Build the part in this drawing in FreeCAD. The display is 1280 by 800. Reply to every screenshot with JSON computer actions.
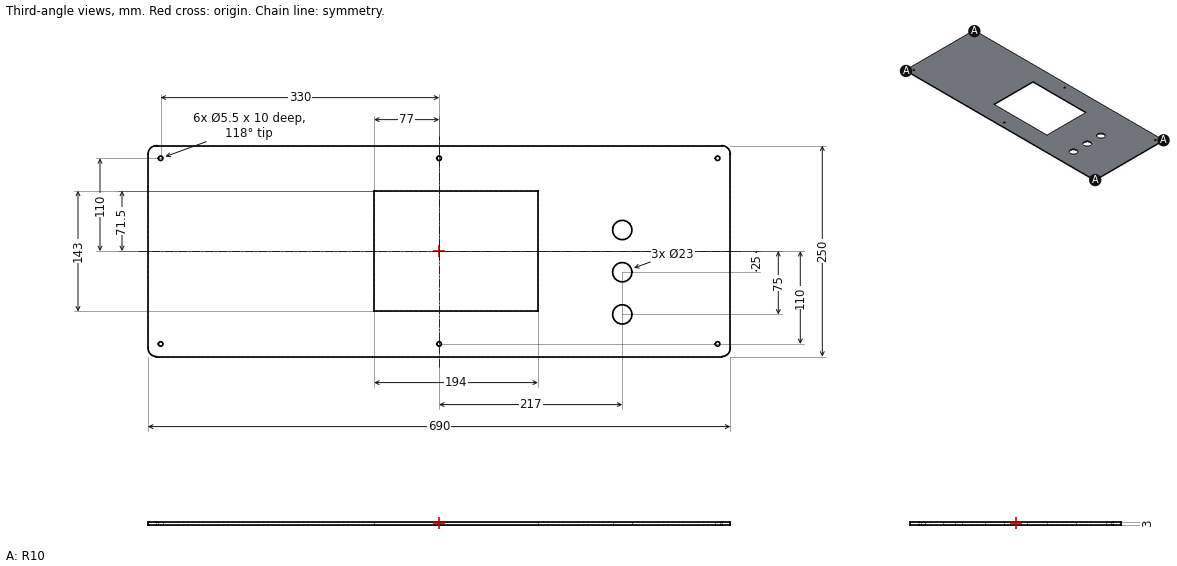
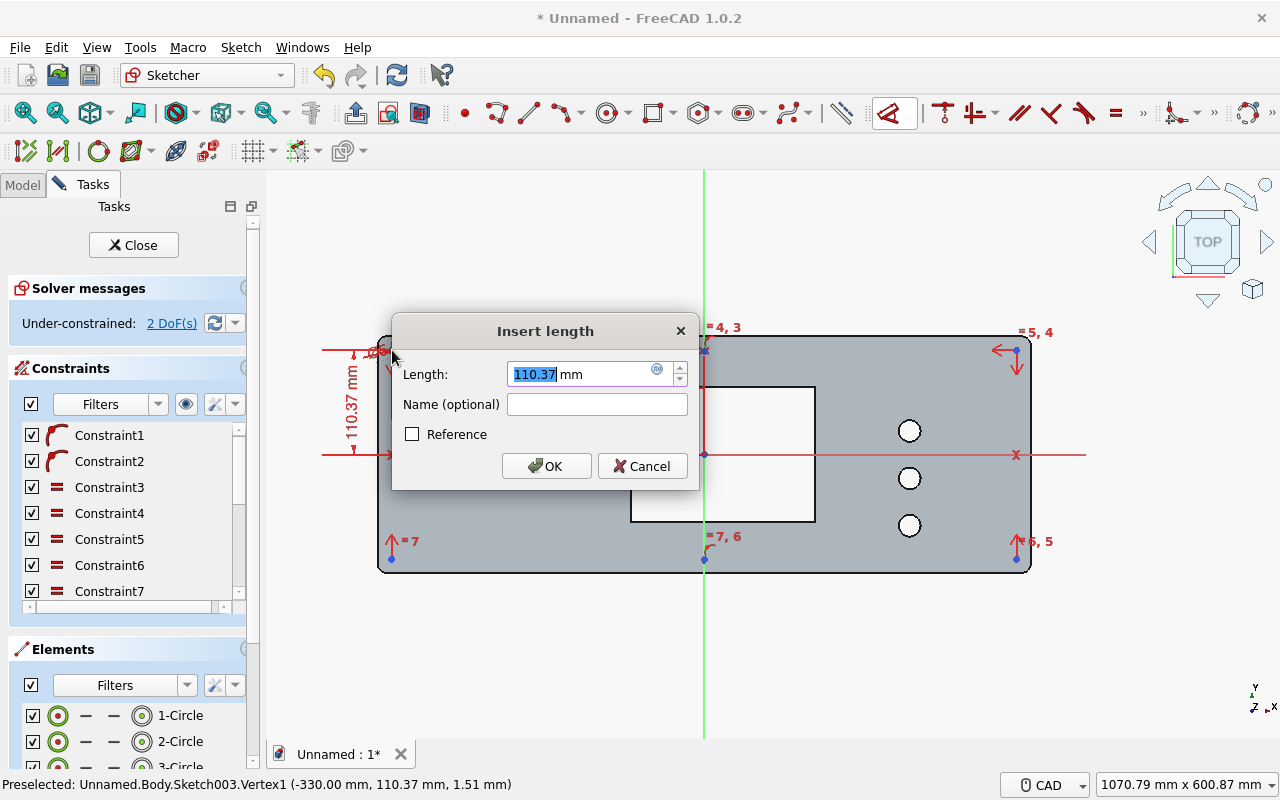
{"action": "type", "text": "110"}
{"action": "key", "text": "Return"}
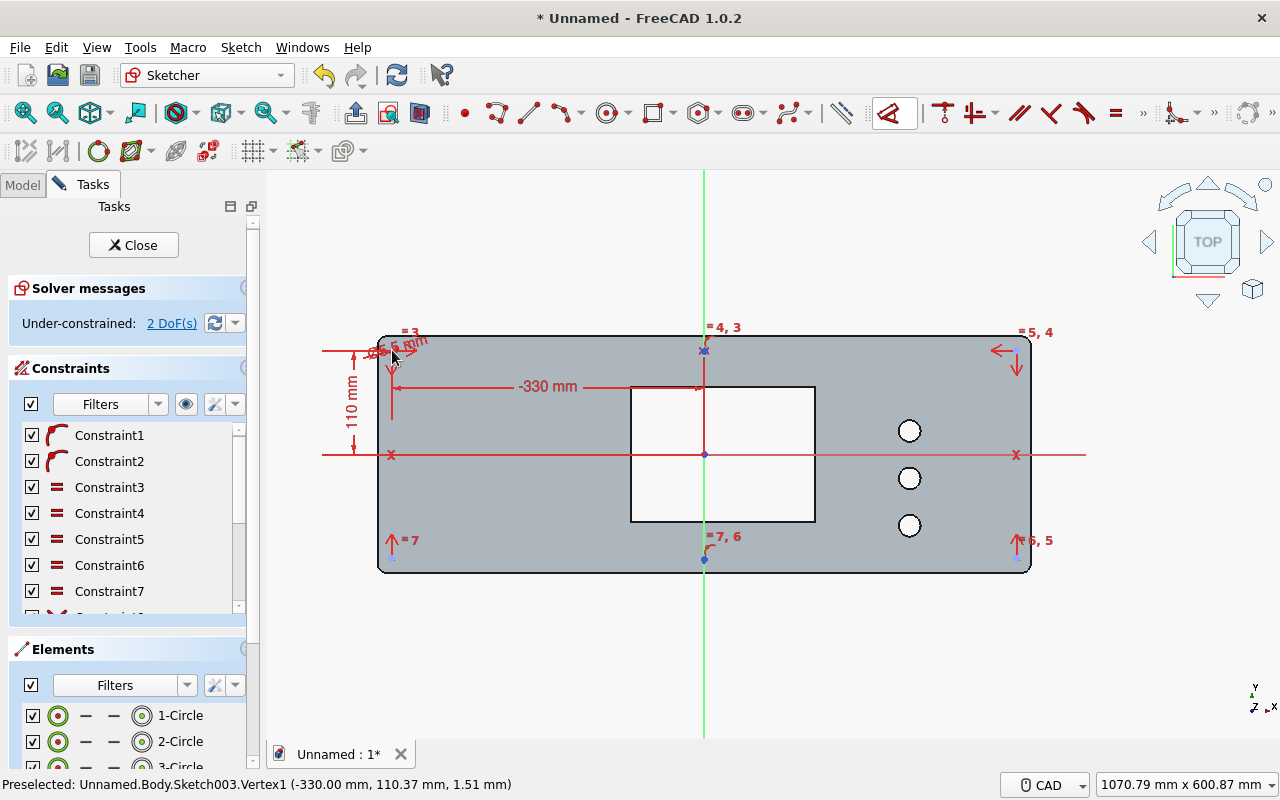
{"action": "left_click", "coordinate": [704, 351]}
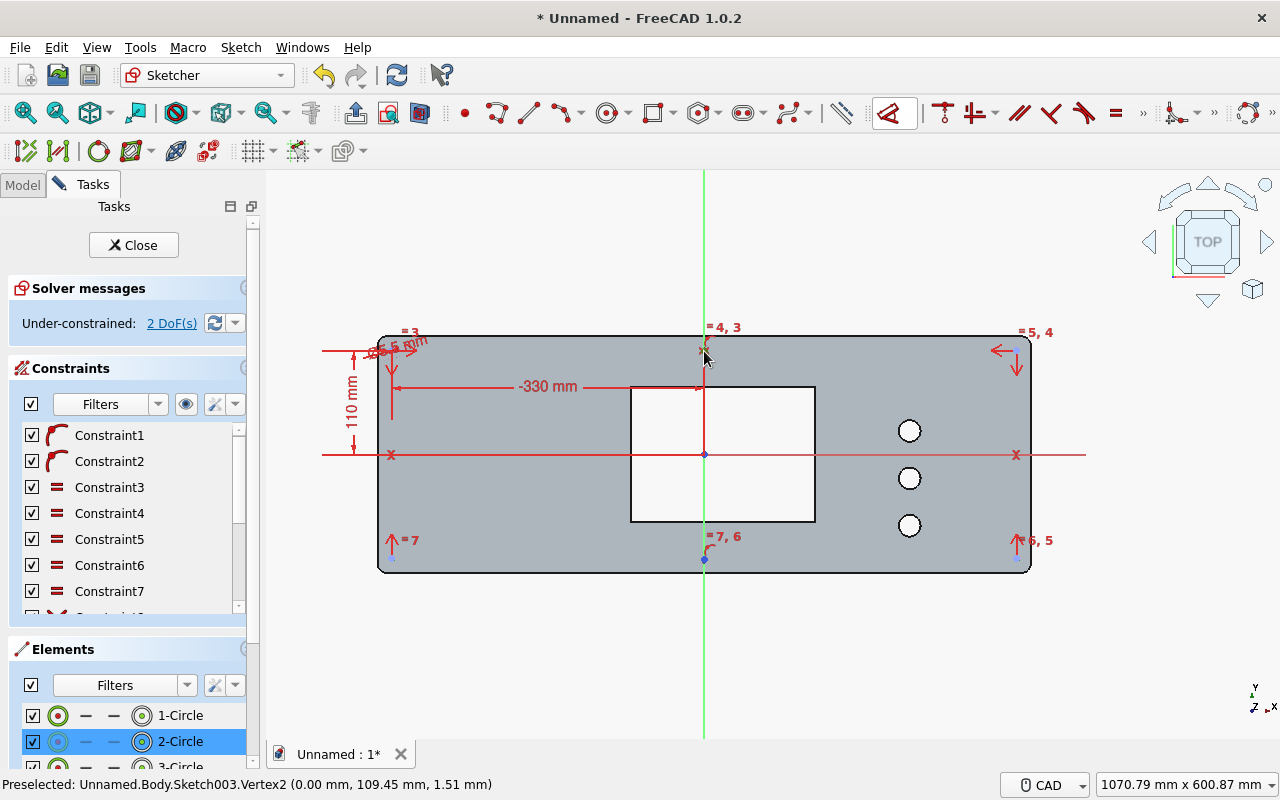
{"action": "left_click", "coordinate": [912, 114]}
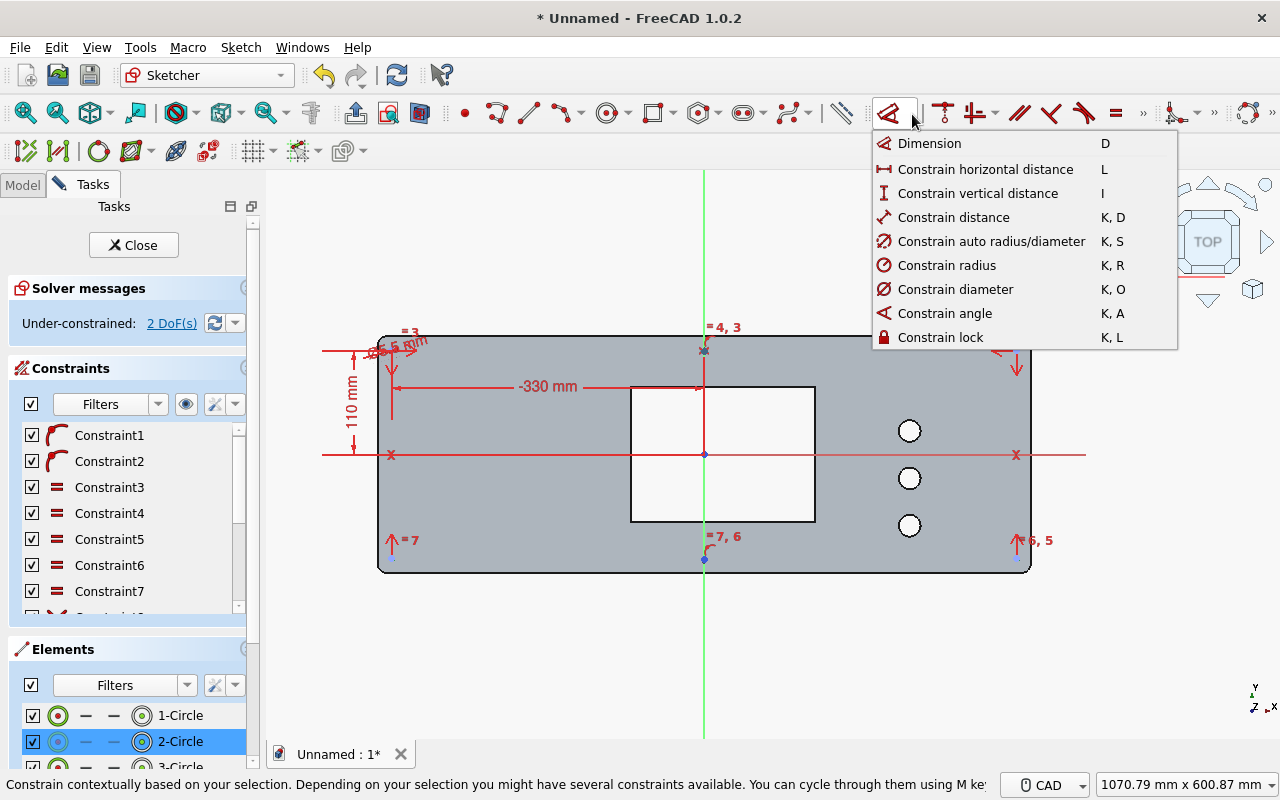
{"action": "left_click", "coordinate": [1025, 193]}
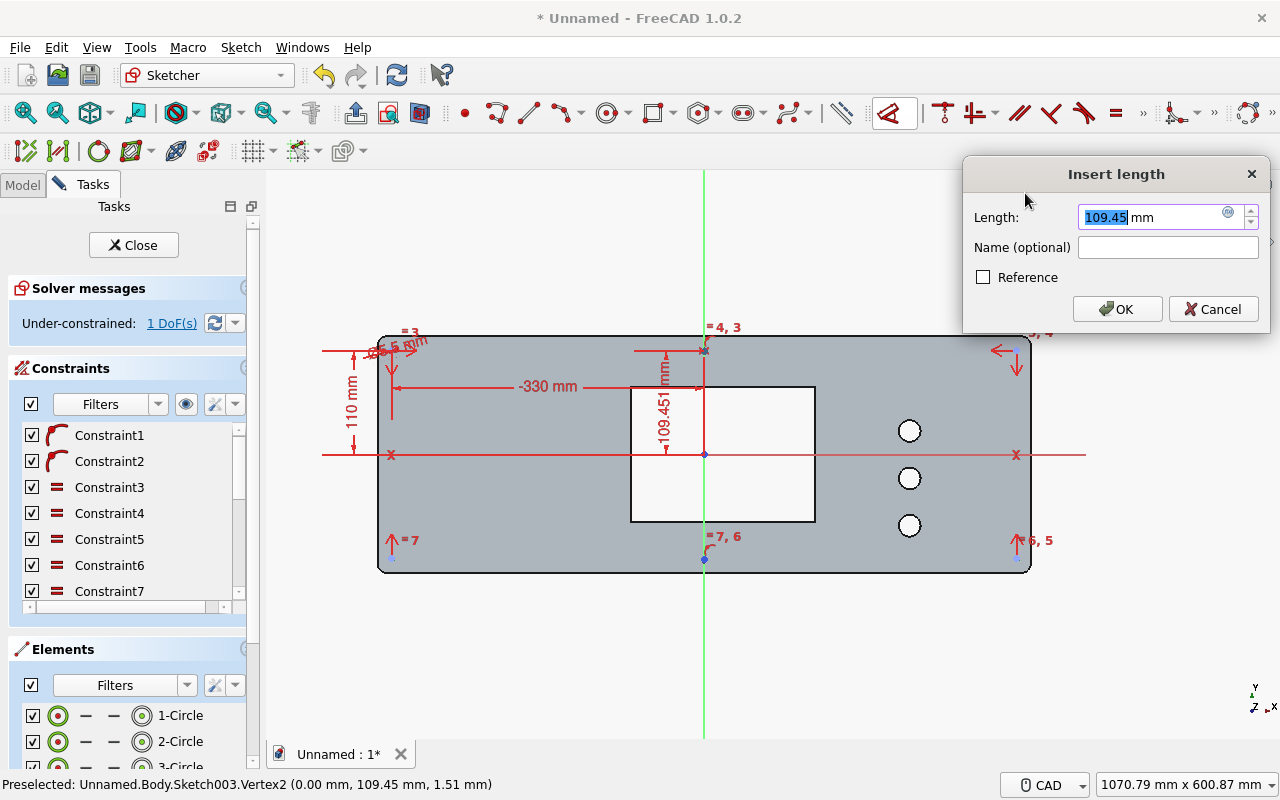
{"action": "type", "text": "110"}
{"action": "key", "text": "Return"}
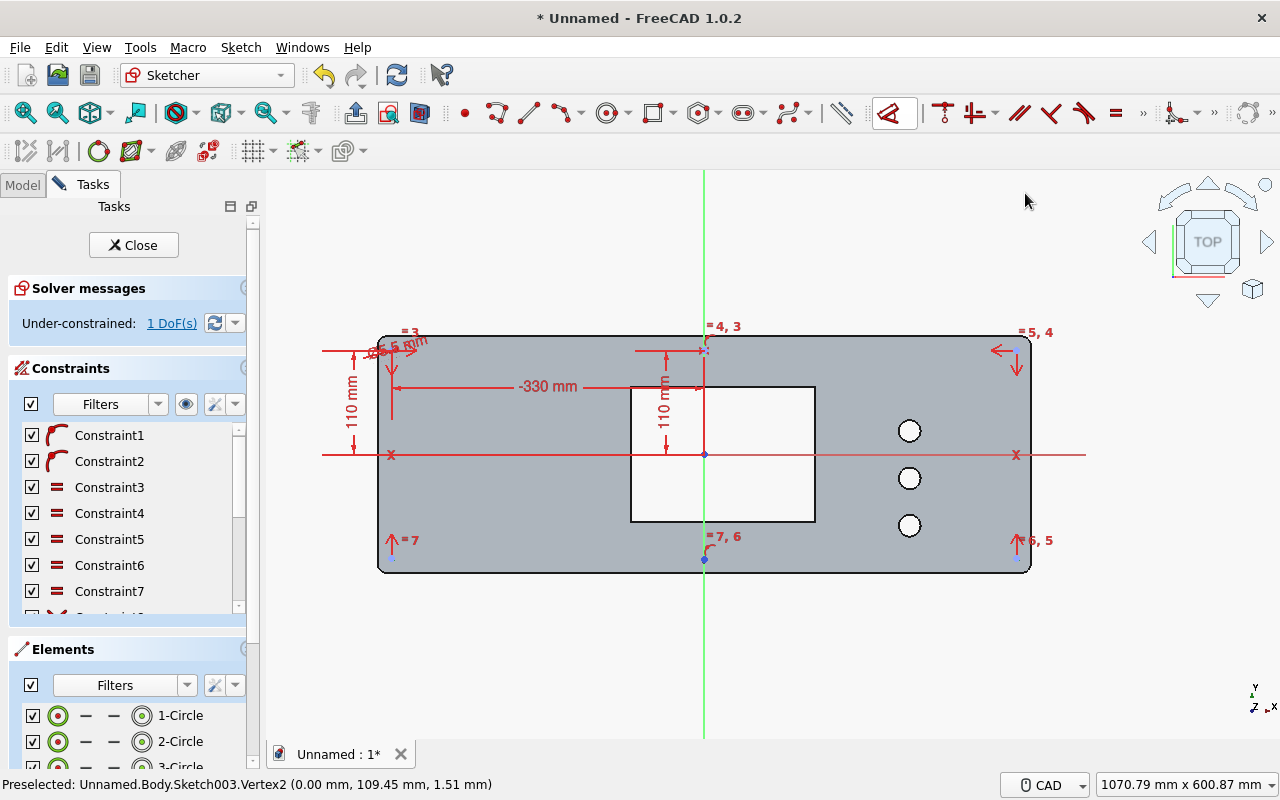
{"action": "left_click", "coordinate": [704, 560]}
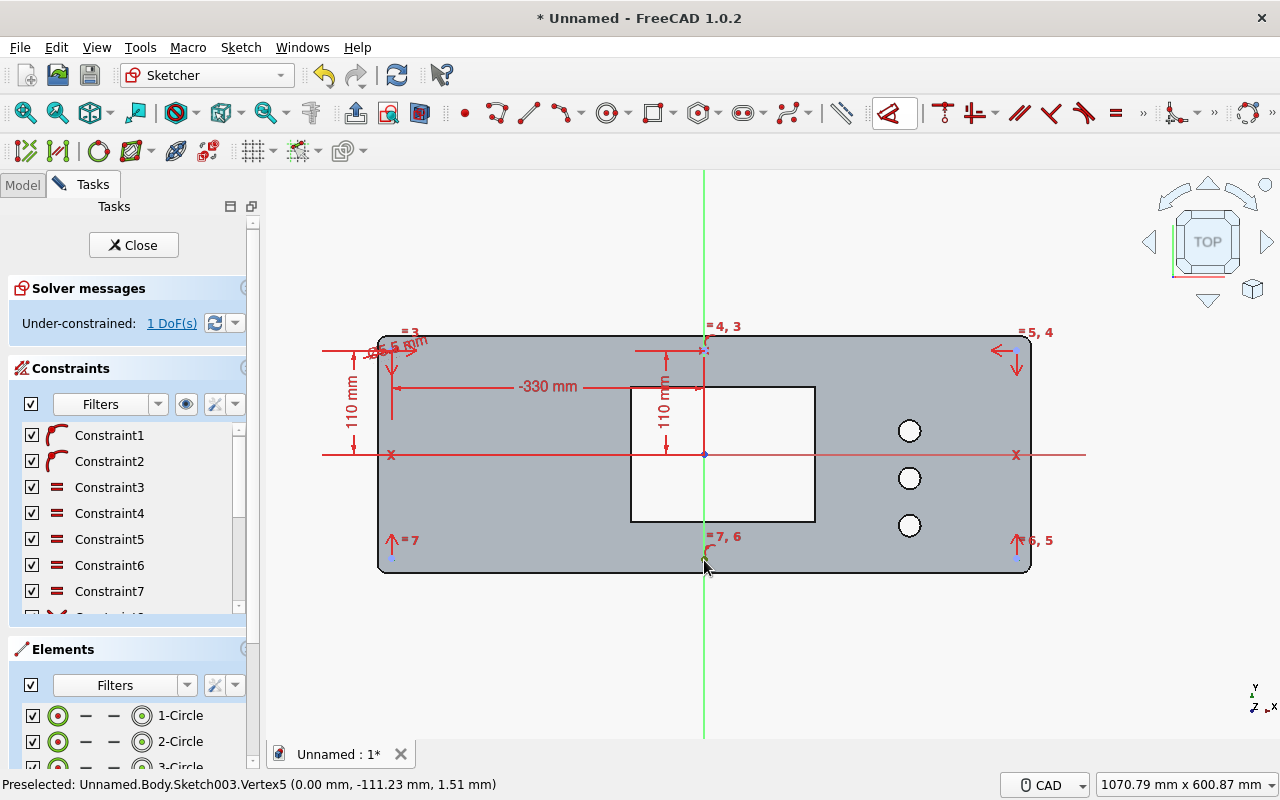
{"action": "left_click", "coordinate": [912, 114]}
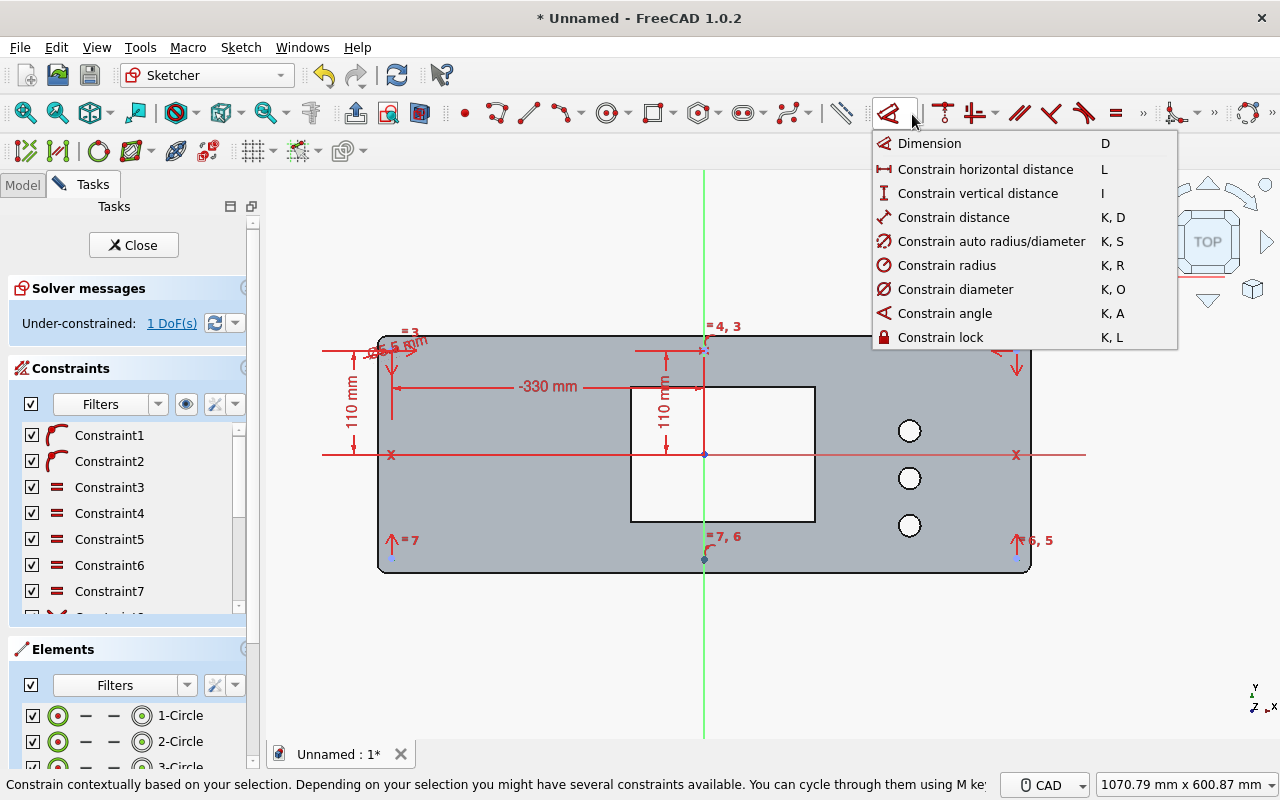
{"action": "left_click", "coordinate": [1025, 193]}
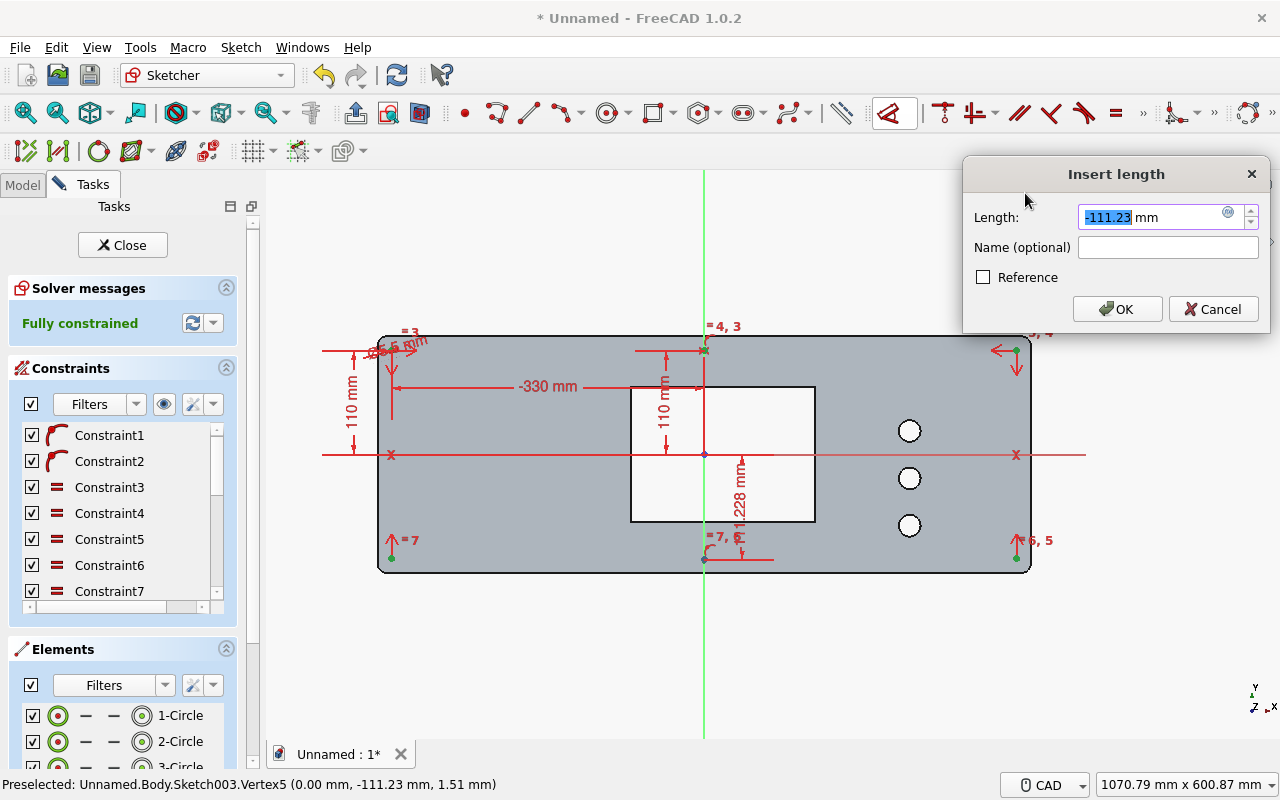
{"action": "type", "text": "-110"}
{"action": "key", "text": "Return"}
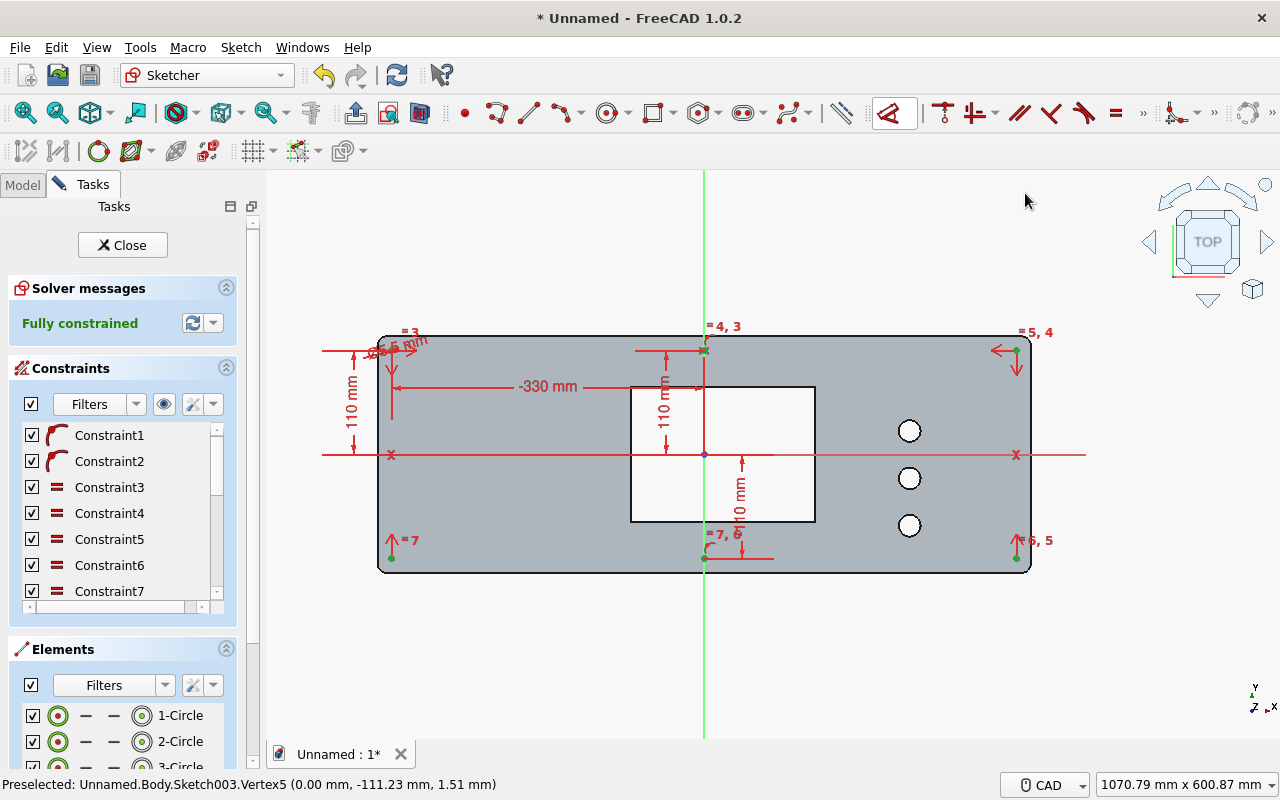
{"action": "left_click", "coordinate": [123, 245]}